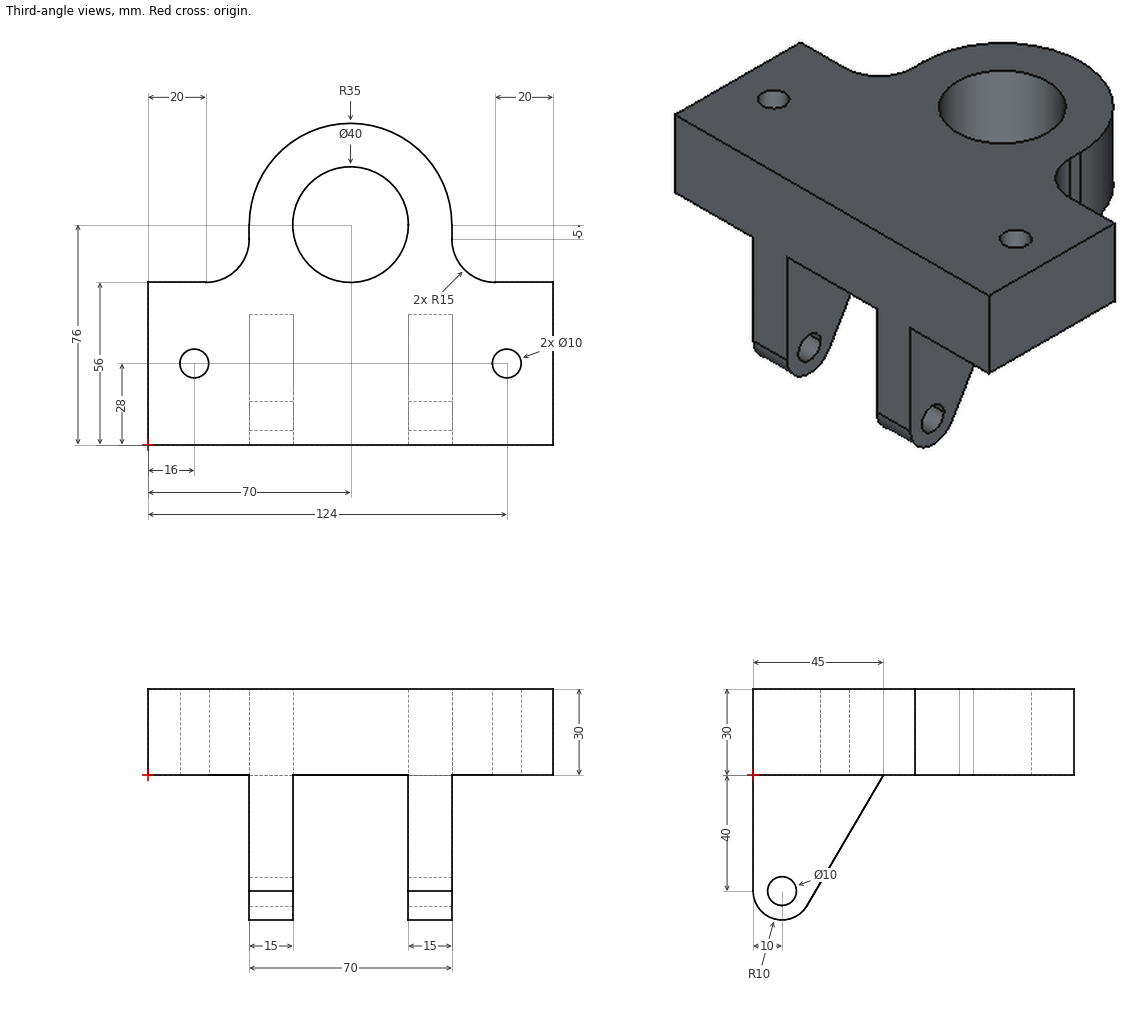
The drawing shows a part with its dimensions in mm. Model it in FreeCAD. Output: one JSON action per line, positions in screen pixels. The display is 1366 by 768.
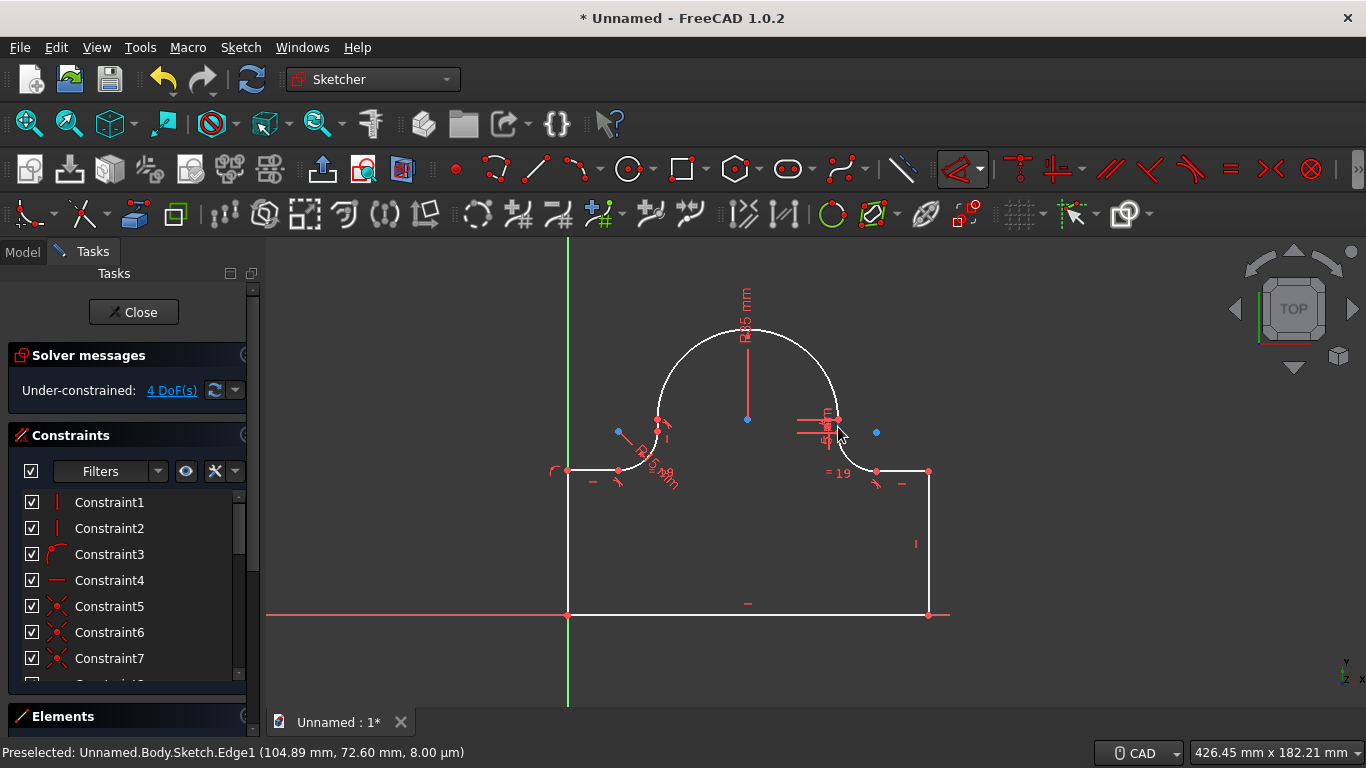
{"action": "scroll", "coordinate": [658, 423], "scroll_direction": "up", "scroll_amount": 7}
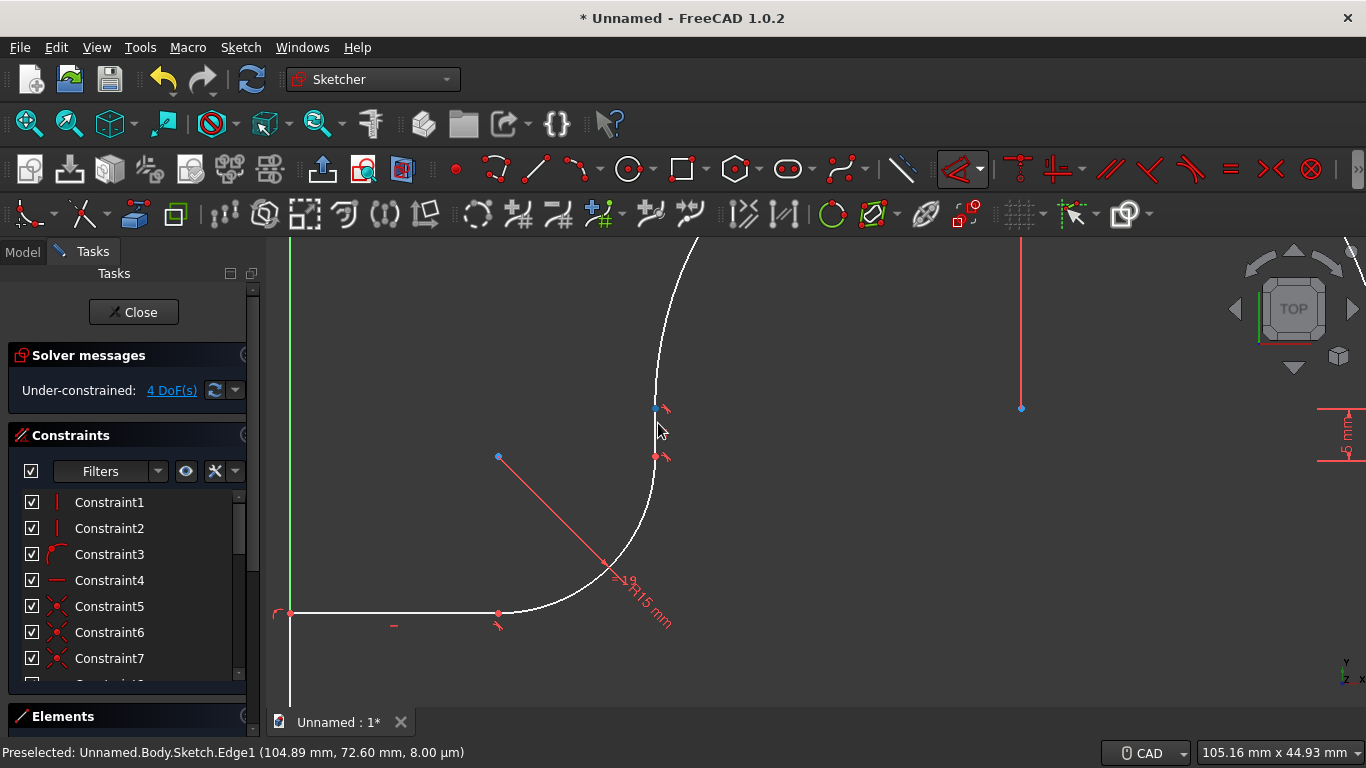
{"action": "left_click", "coordinate": [655, 423]}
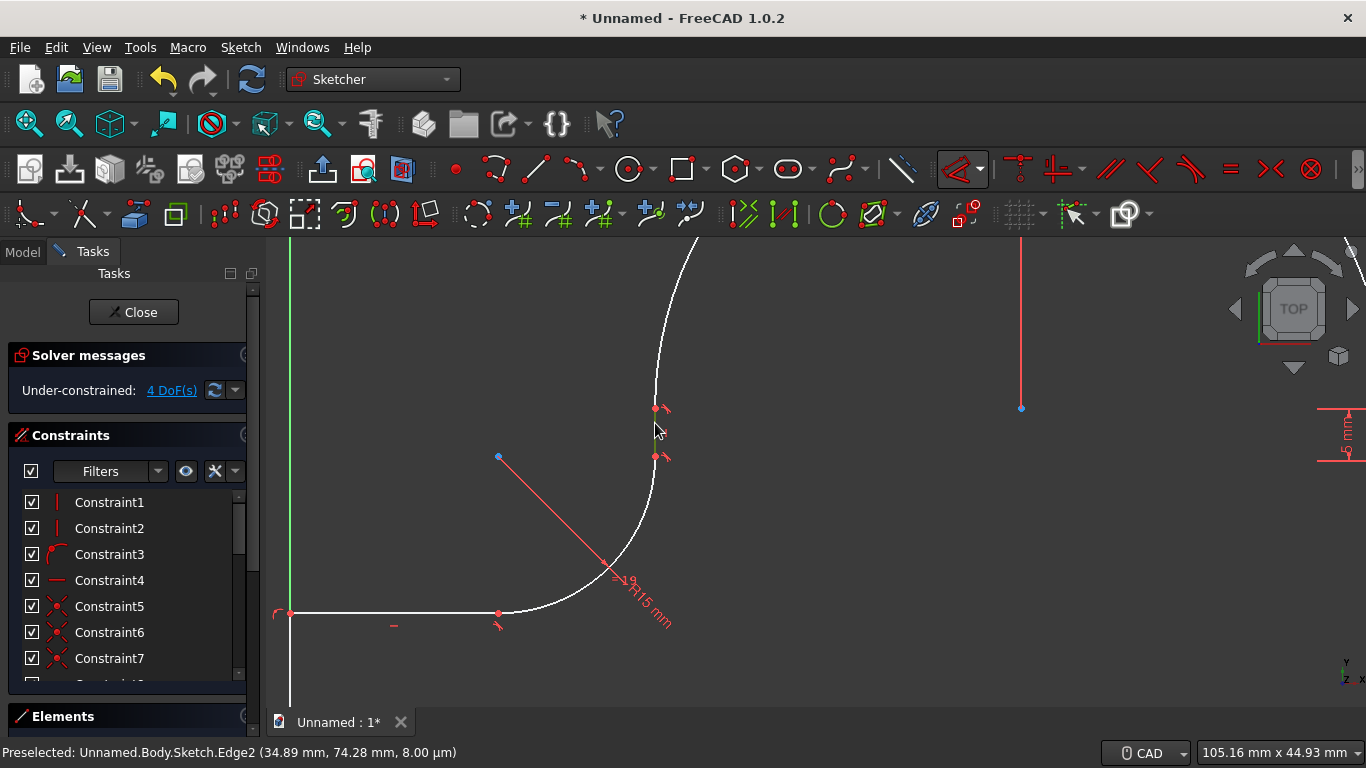
{"action": "left_click", "coordinate": [982, 170]}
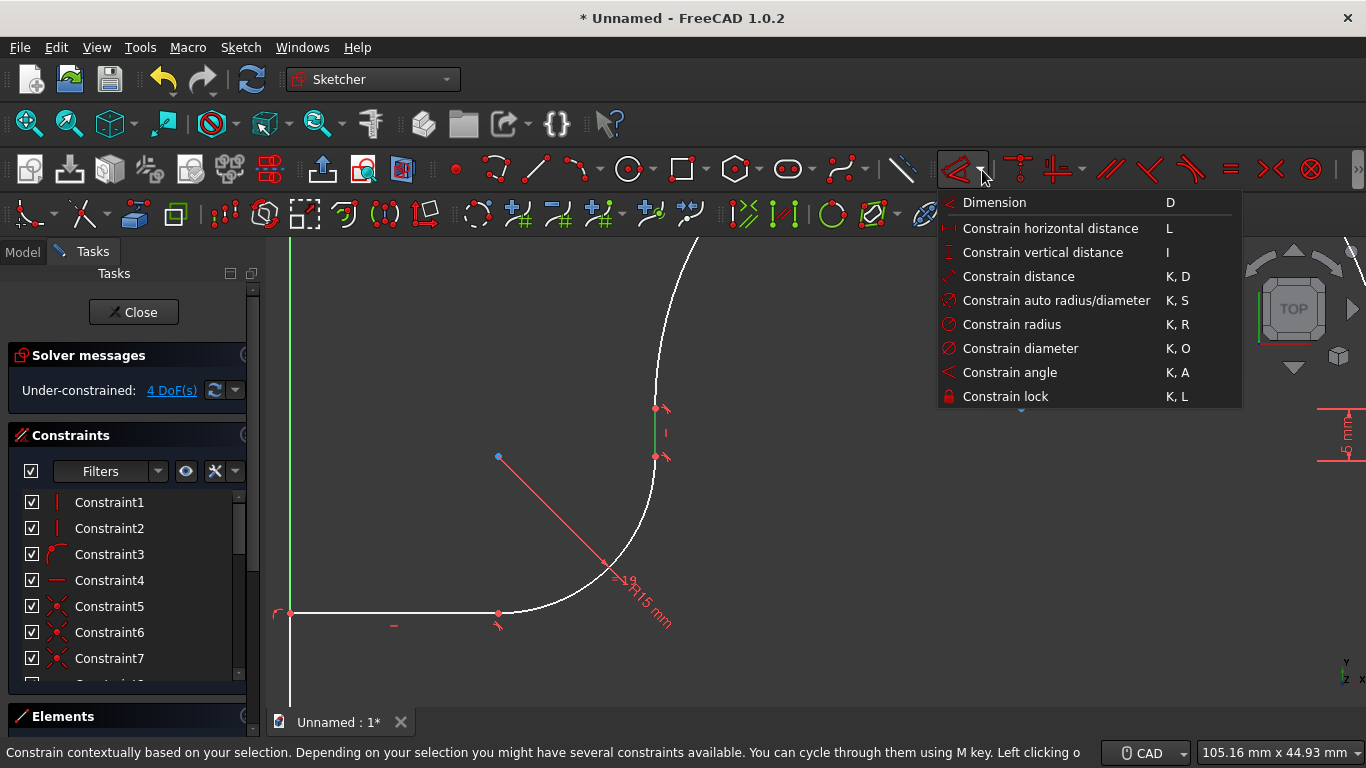
{"action": "left_click", "coordinate": [1090, 252]}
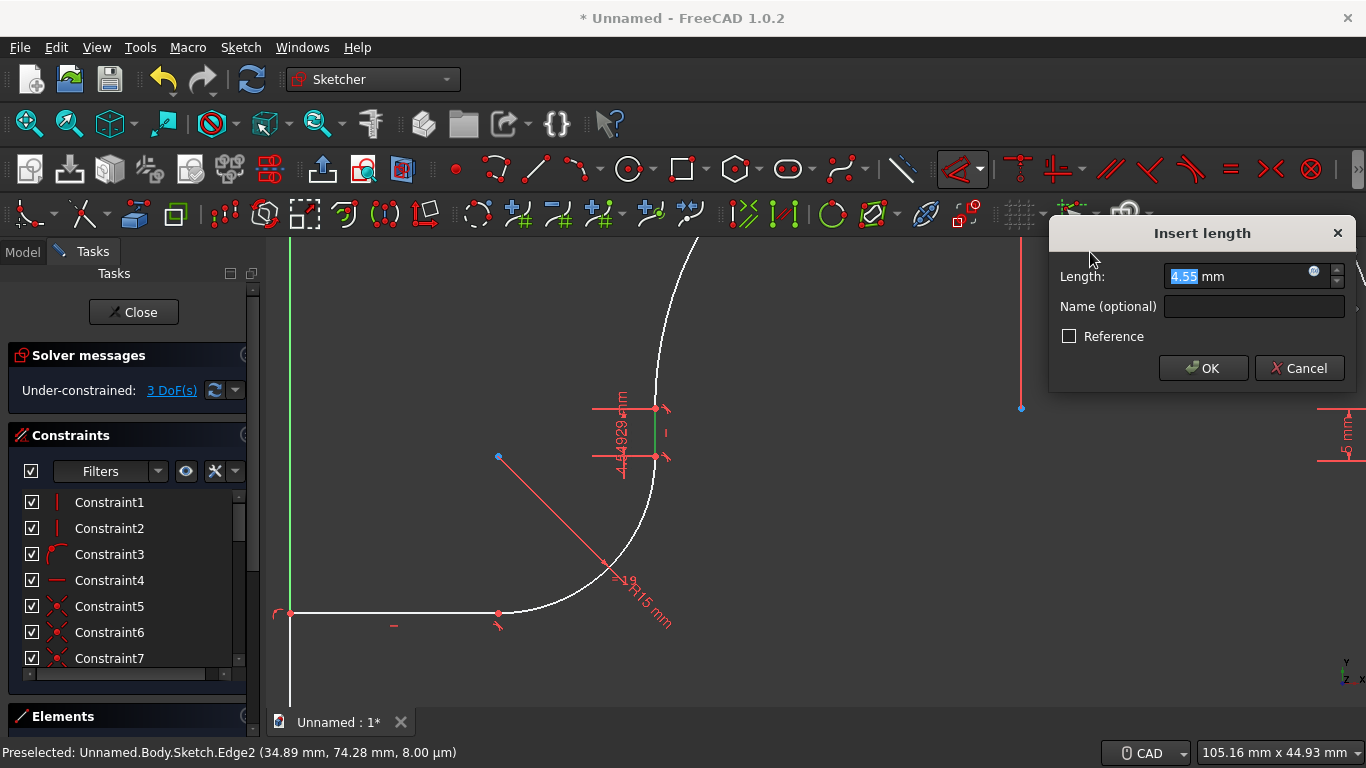
{"action": "type", "text": "5"}
{"action": "key", "text": "Return"}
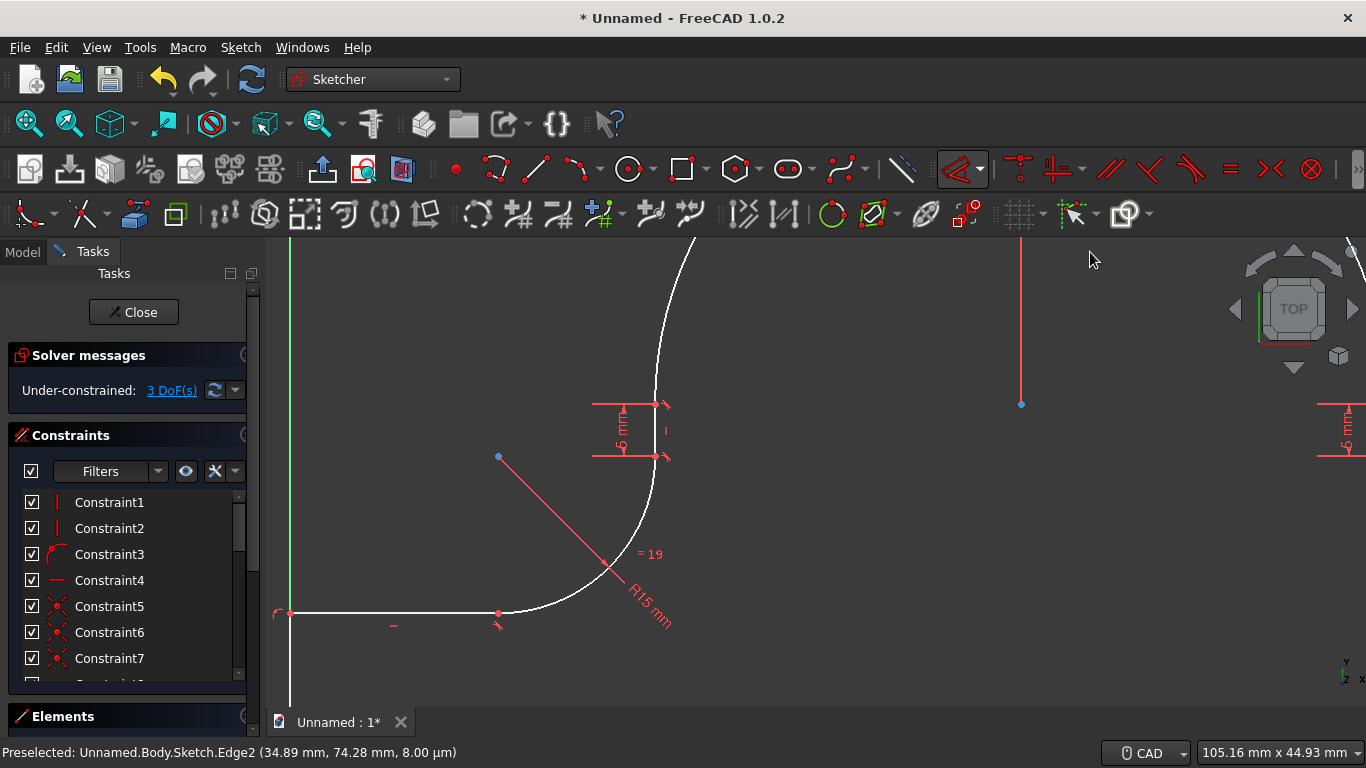
{"action": "scroll", "coordinate": [658, 423], "scroll_direction": "down", "scroll_amount": 7}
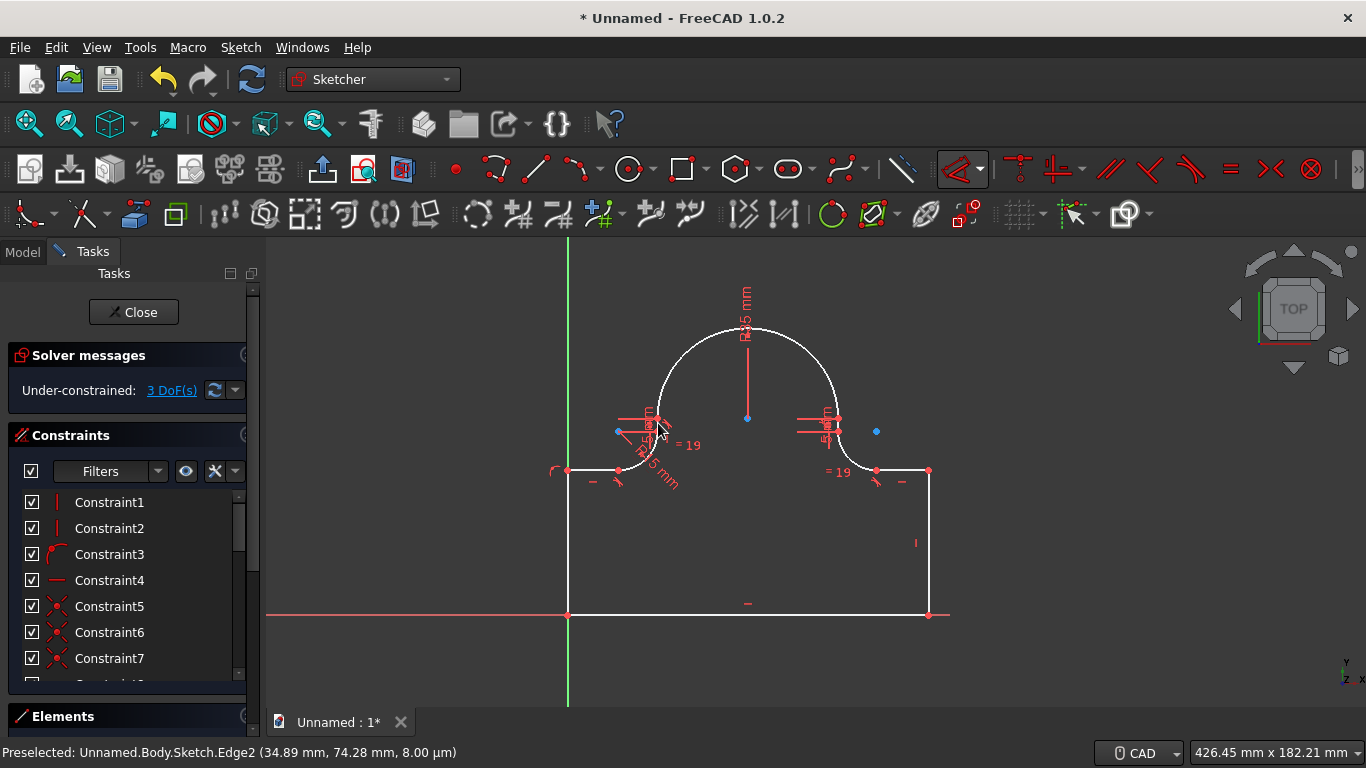
{"action": "left_click", "coordinate": [603, 470]}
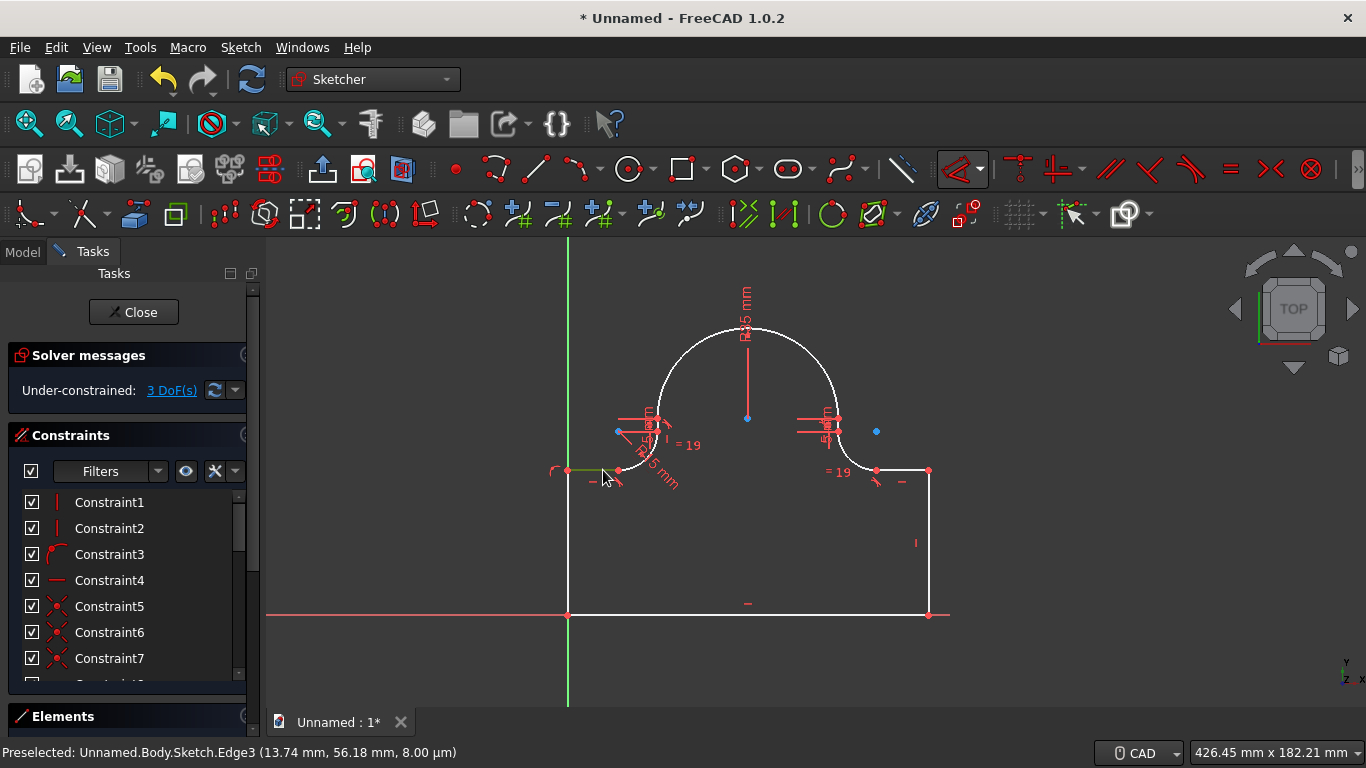
{"action": "key", "text": "l"}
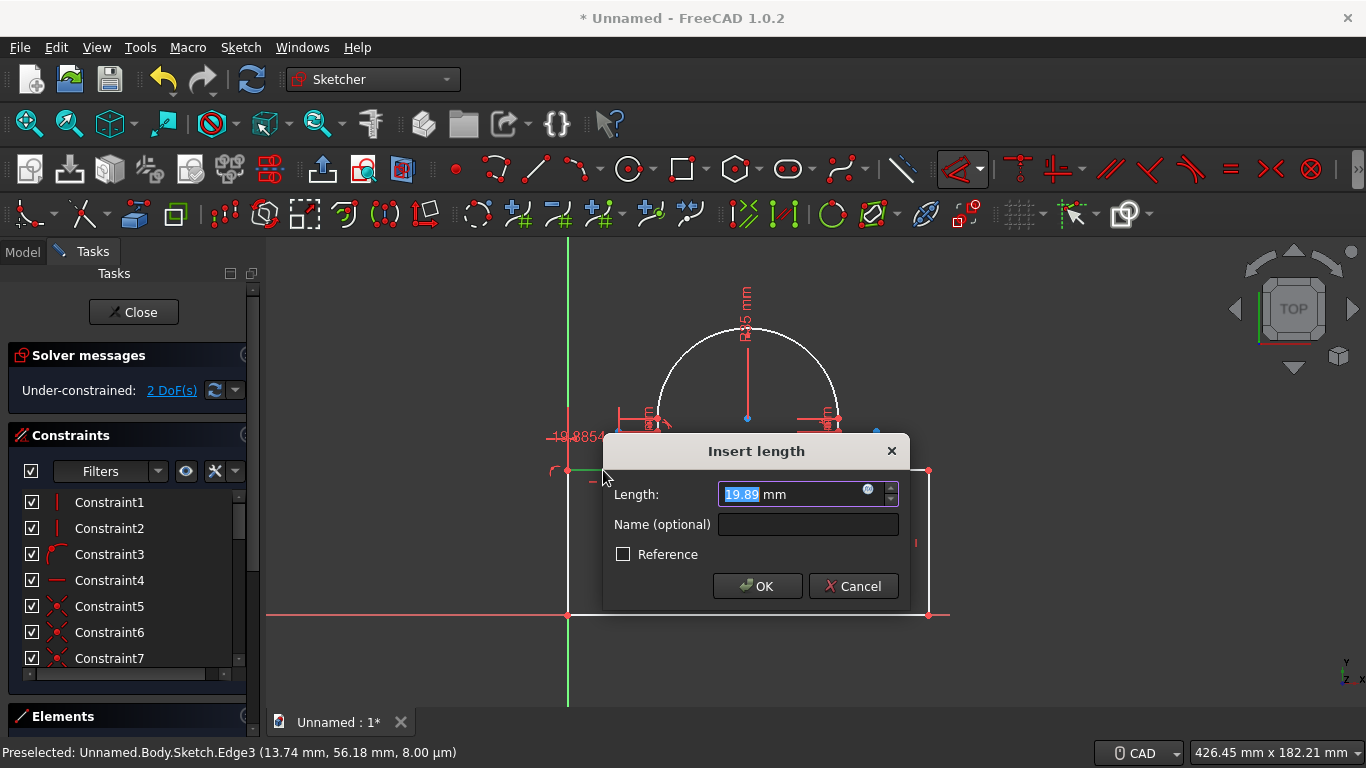
{"action": "type", "text": "20"}
{"action": "key", "text": "Return"}